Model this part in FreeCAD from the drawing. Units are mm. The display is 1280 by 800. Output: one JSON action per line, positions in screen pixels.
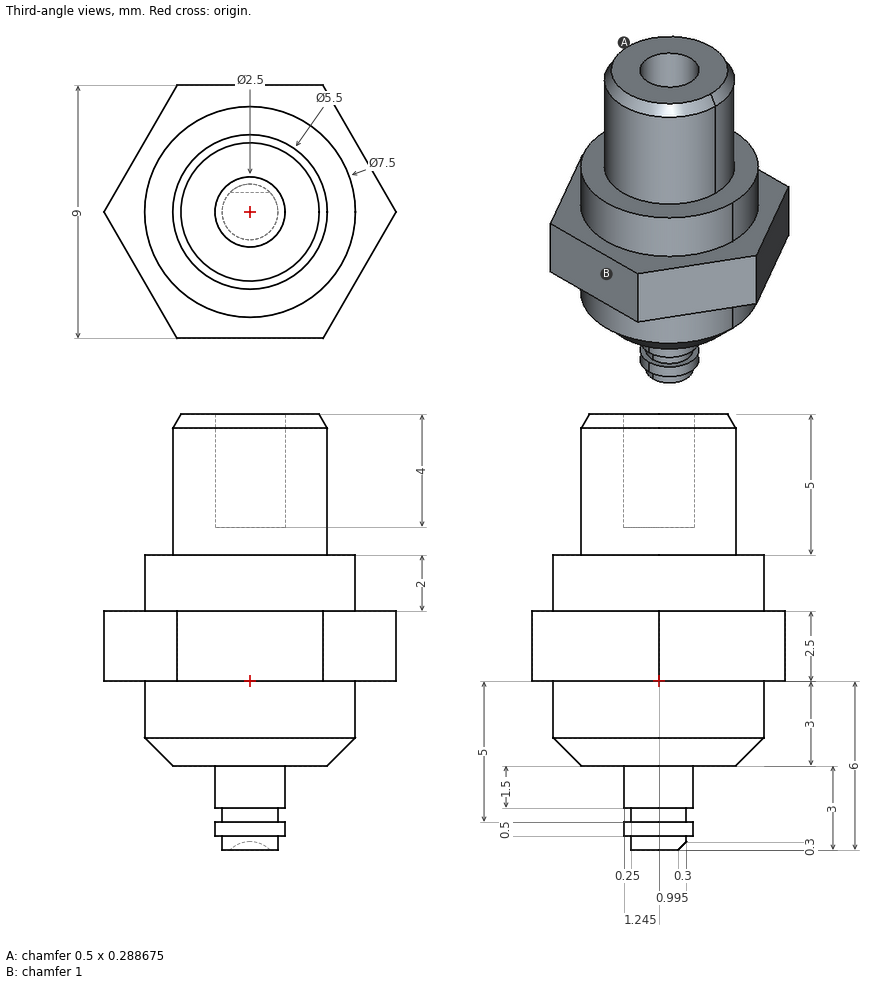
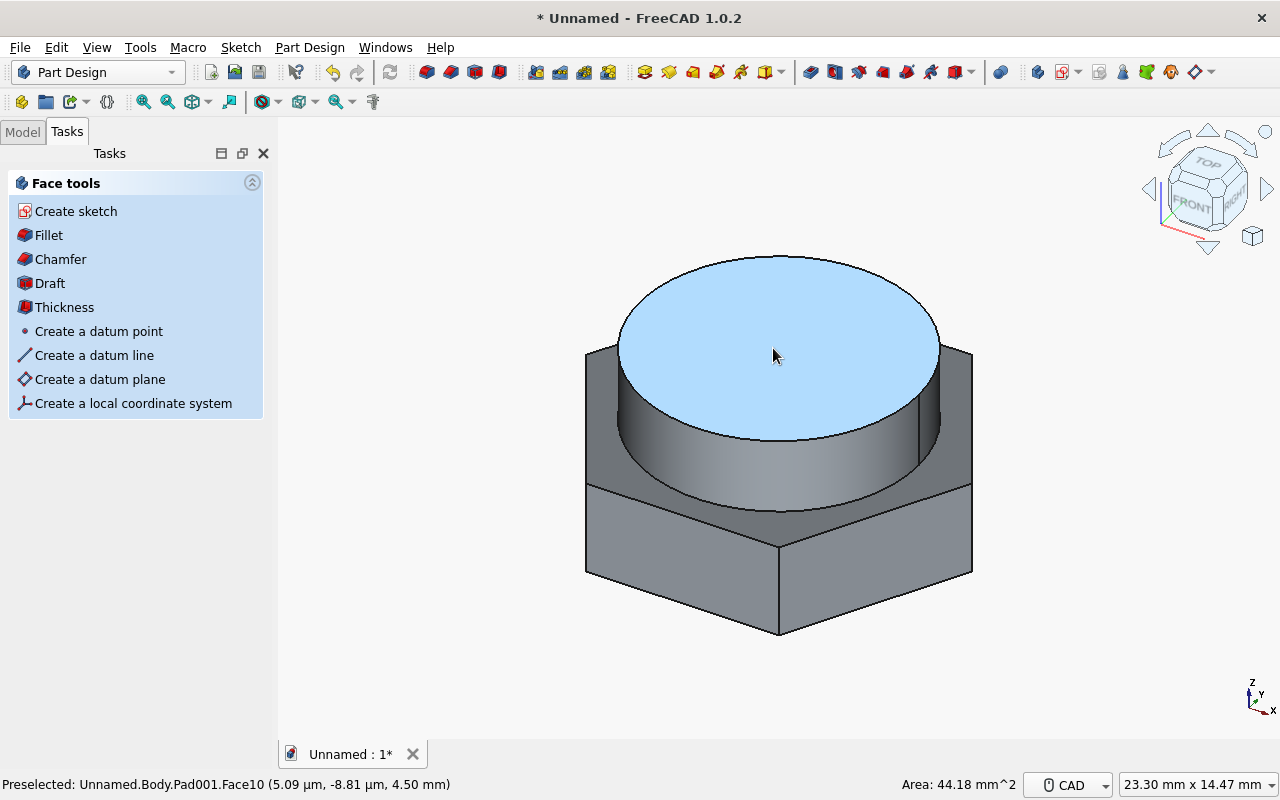
{"action": "left_click", "coordinate": [1062, 72]}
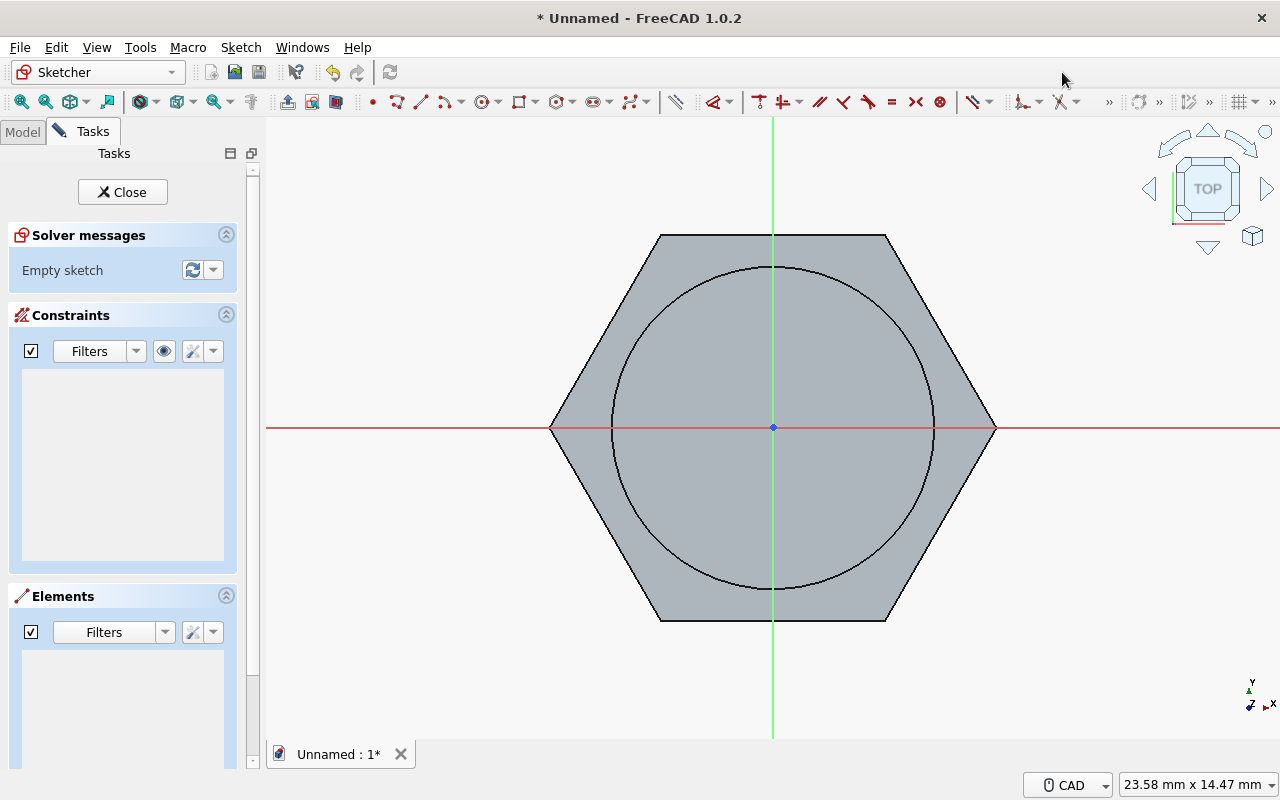
{"action": "scroll", "coordinate": [856, 428], "scroll_direction": "up", "scroll_amount": 3}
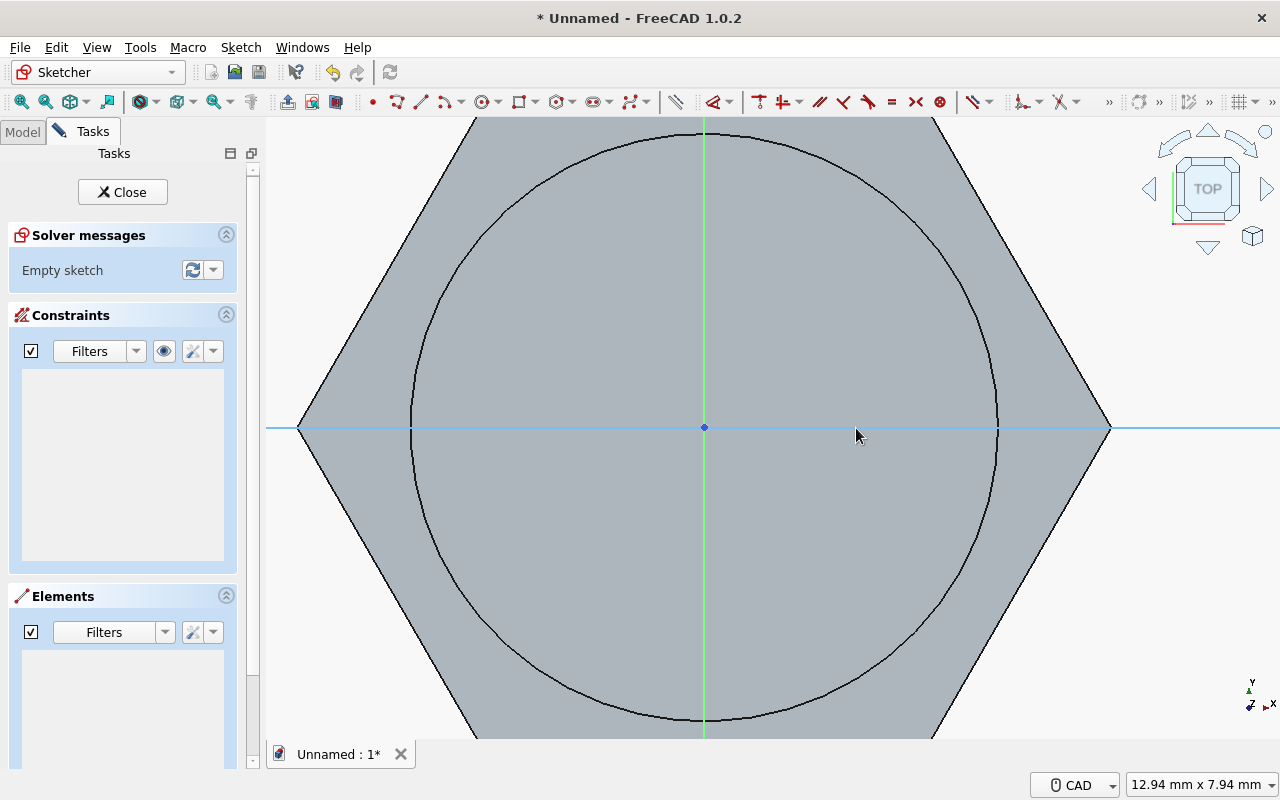
{"action": "left_click", "coordinate": [482, 102]}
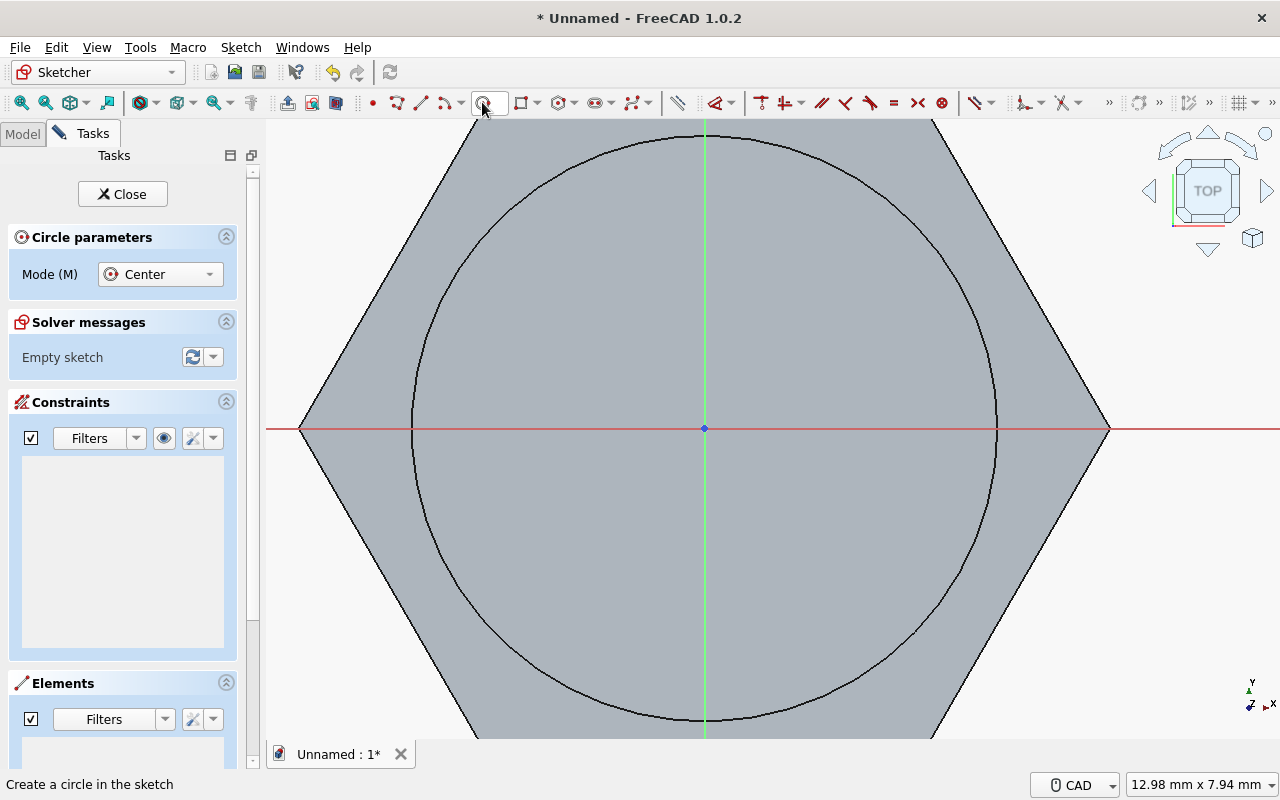
{"action": "left_click", "coordinate": [705, 429]}
{"action": "left_click", "coordinate": [856, 277]}
{"action": "key", "text": "Escape"}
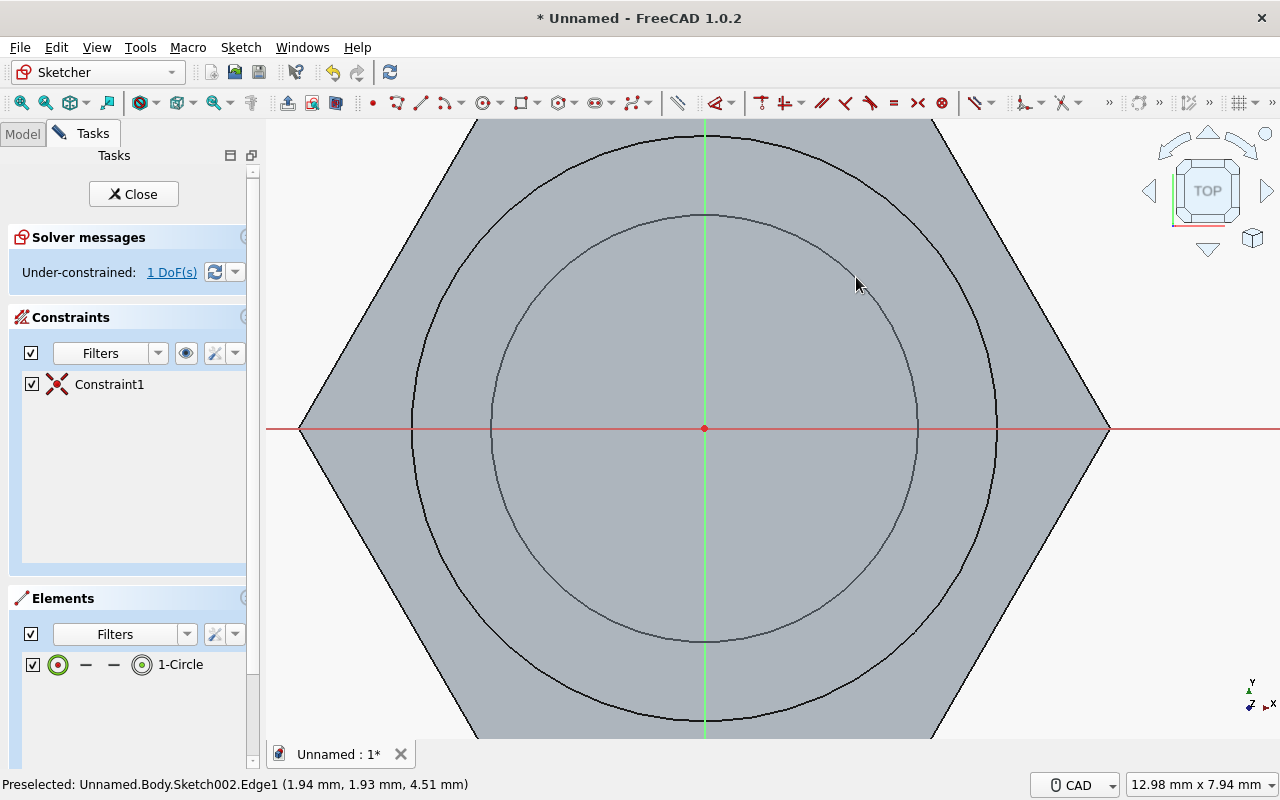
{"action": "left_click", "coordinate": [855, 277]}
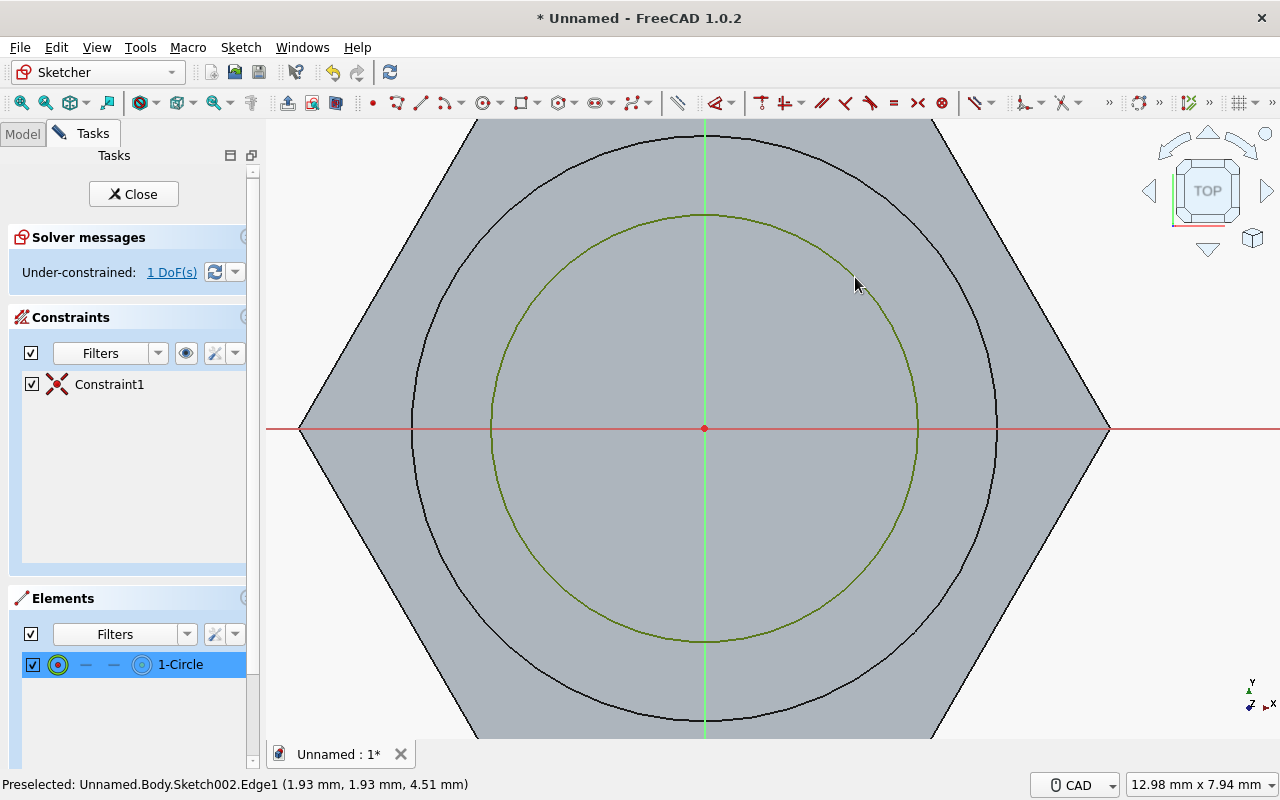
{"action": "key", "text": "k o"}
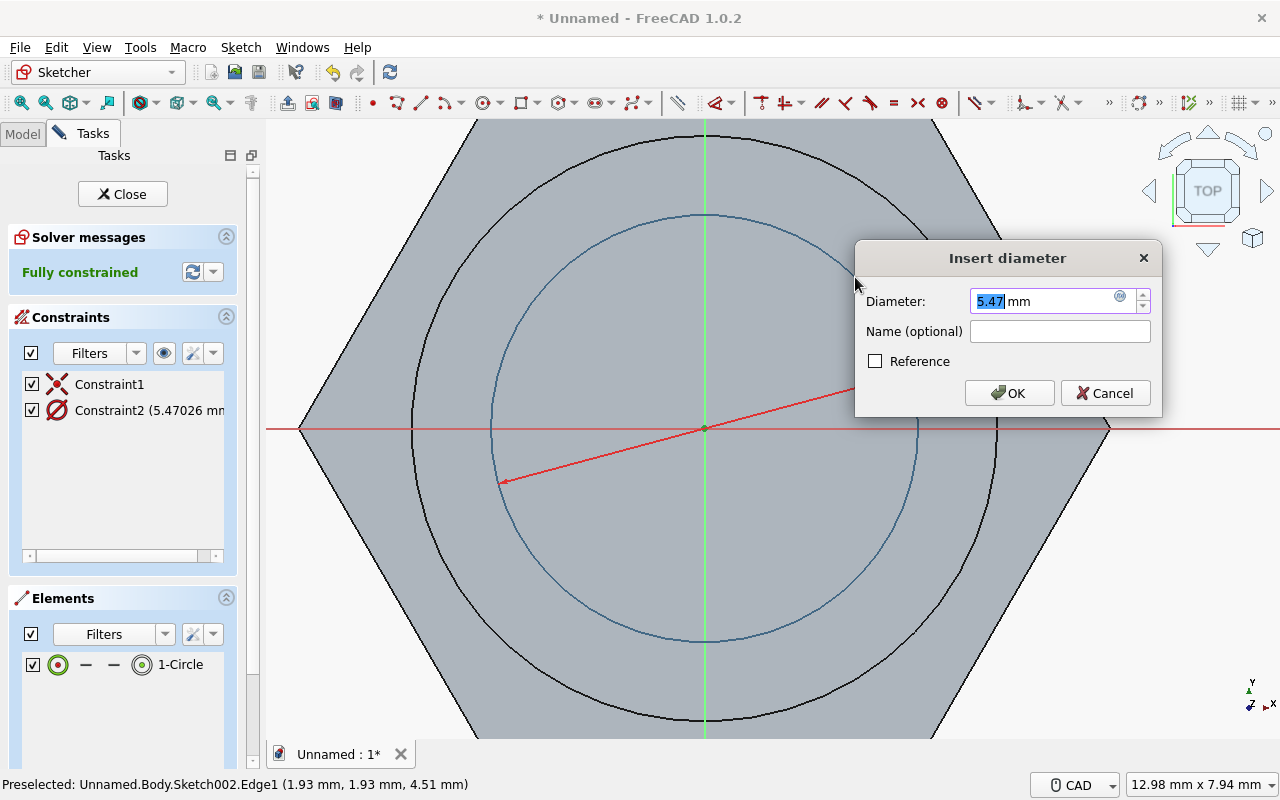
{"action": "type", "text": "5.5"}
{"action": "key", "text": "Return"}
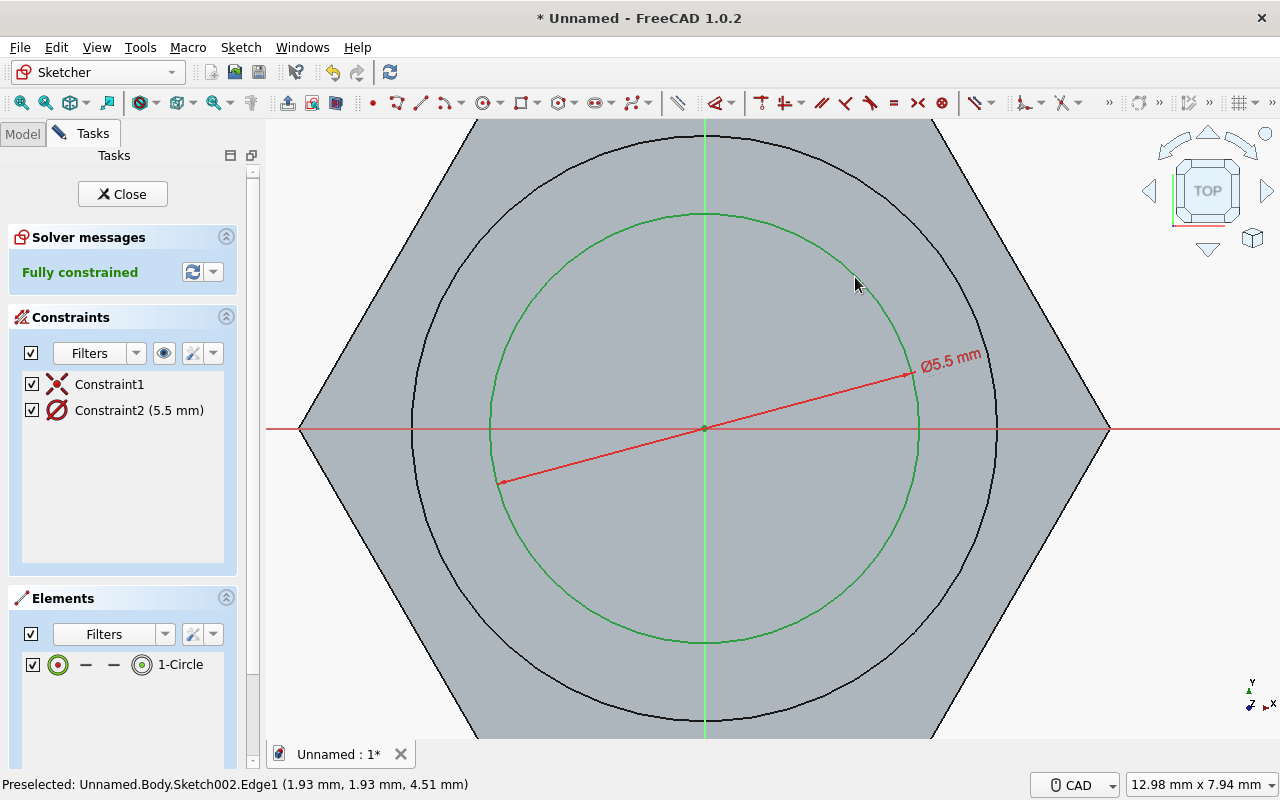
{"action": "left_click", "coordinate": [123, 194]}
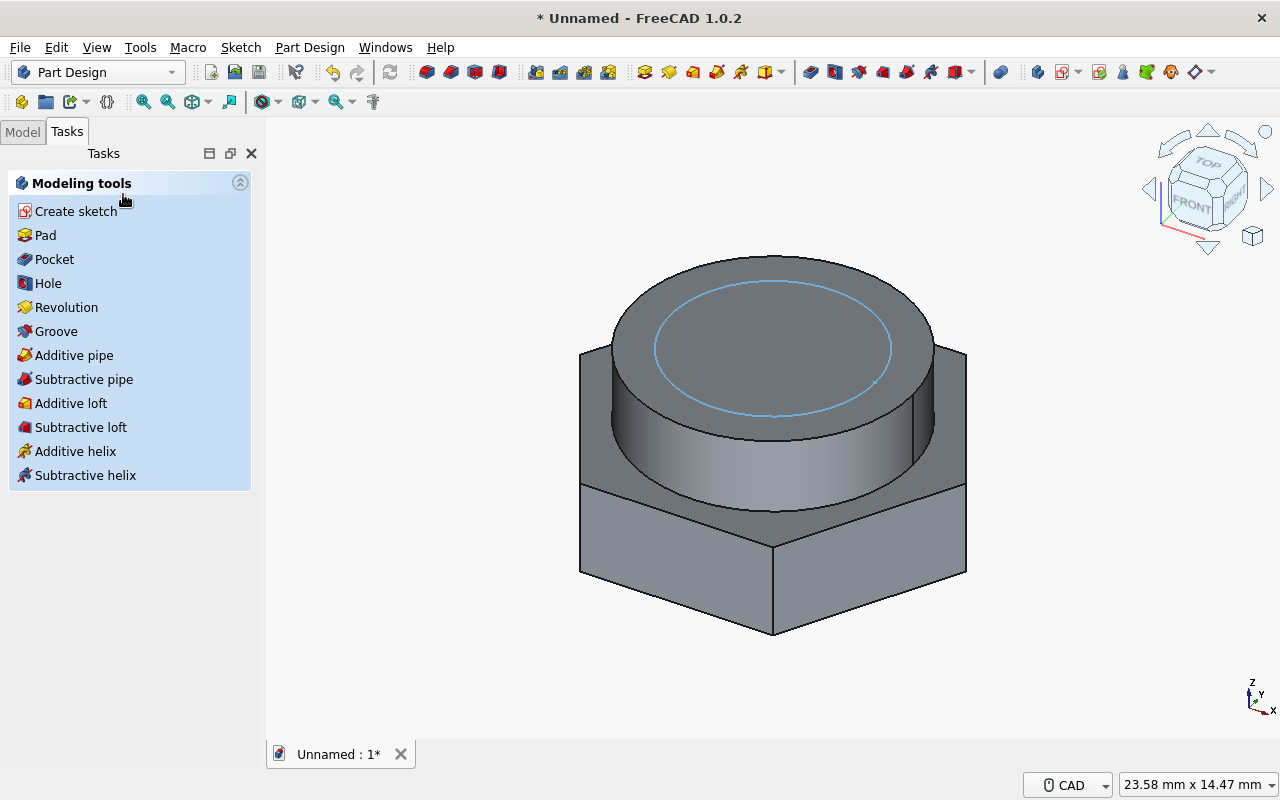
{"action": "left_click", "coordinate": [646, 72]}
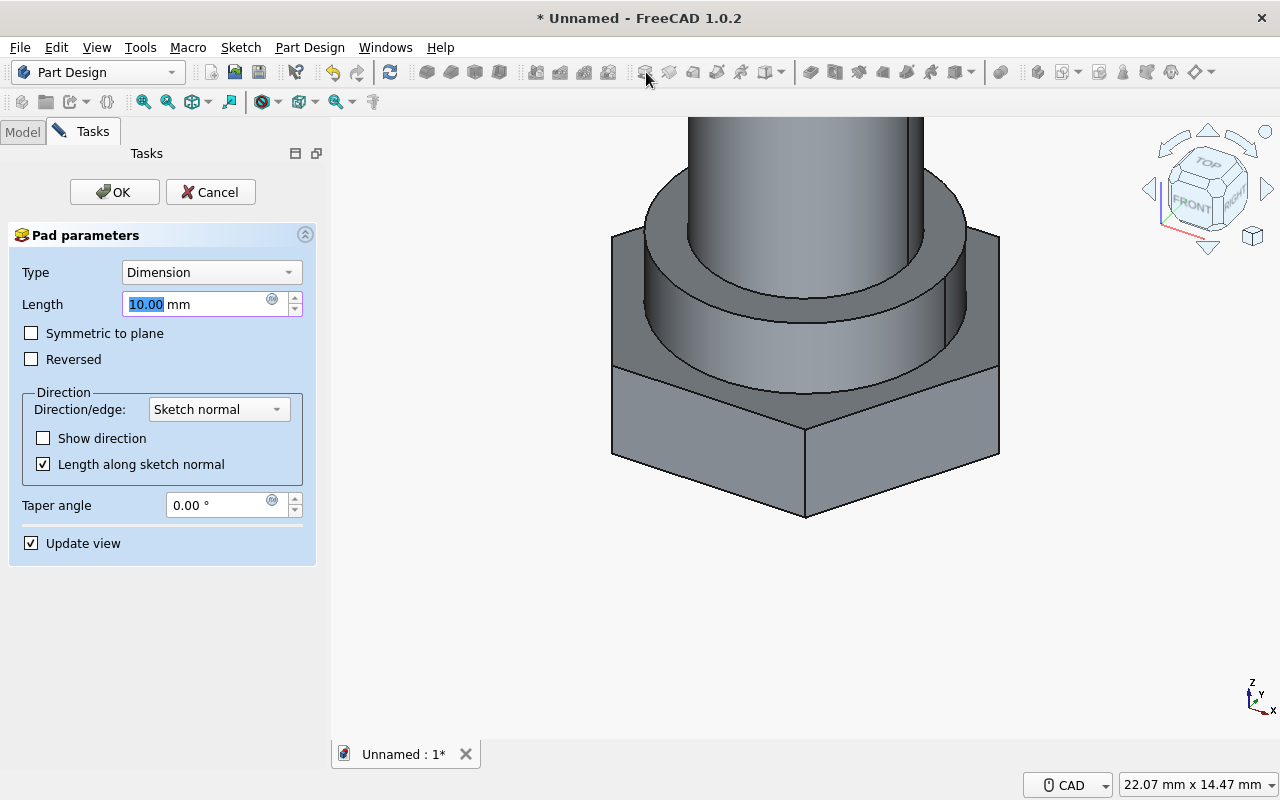
{"action": "type", "text": "5"}
{"action": "key", "text": "Tab"}